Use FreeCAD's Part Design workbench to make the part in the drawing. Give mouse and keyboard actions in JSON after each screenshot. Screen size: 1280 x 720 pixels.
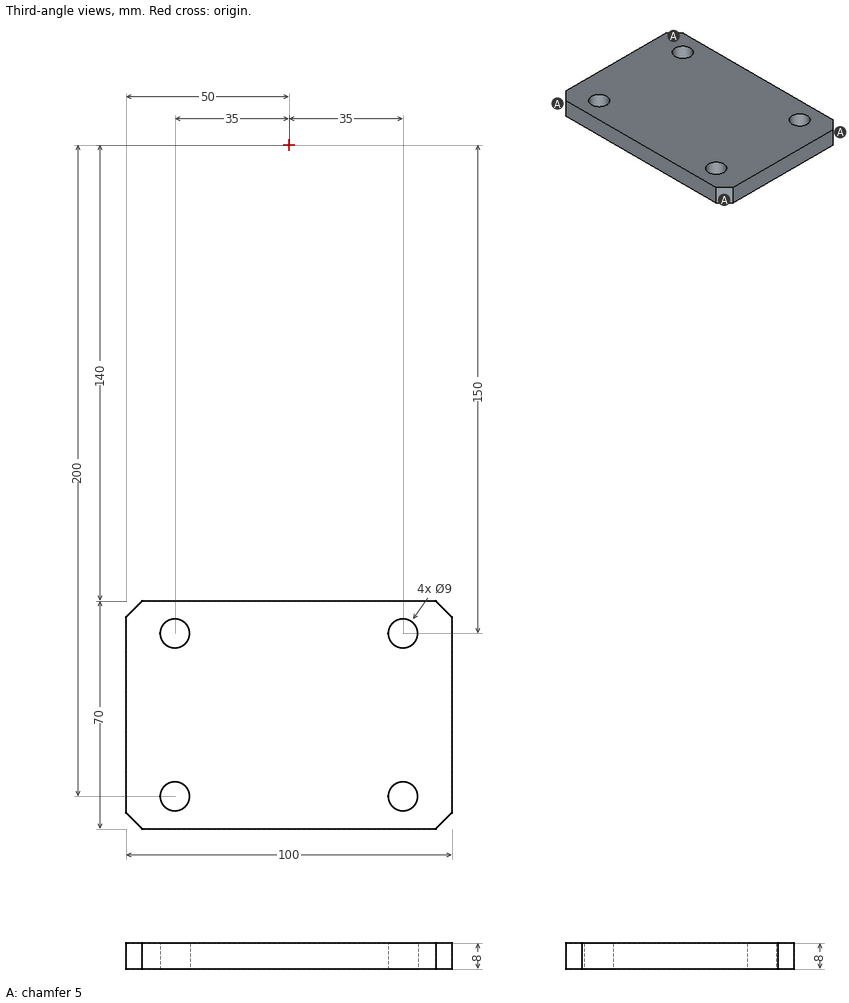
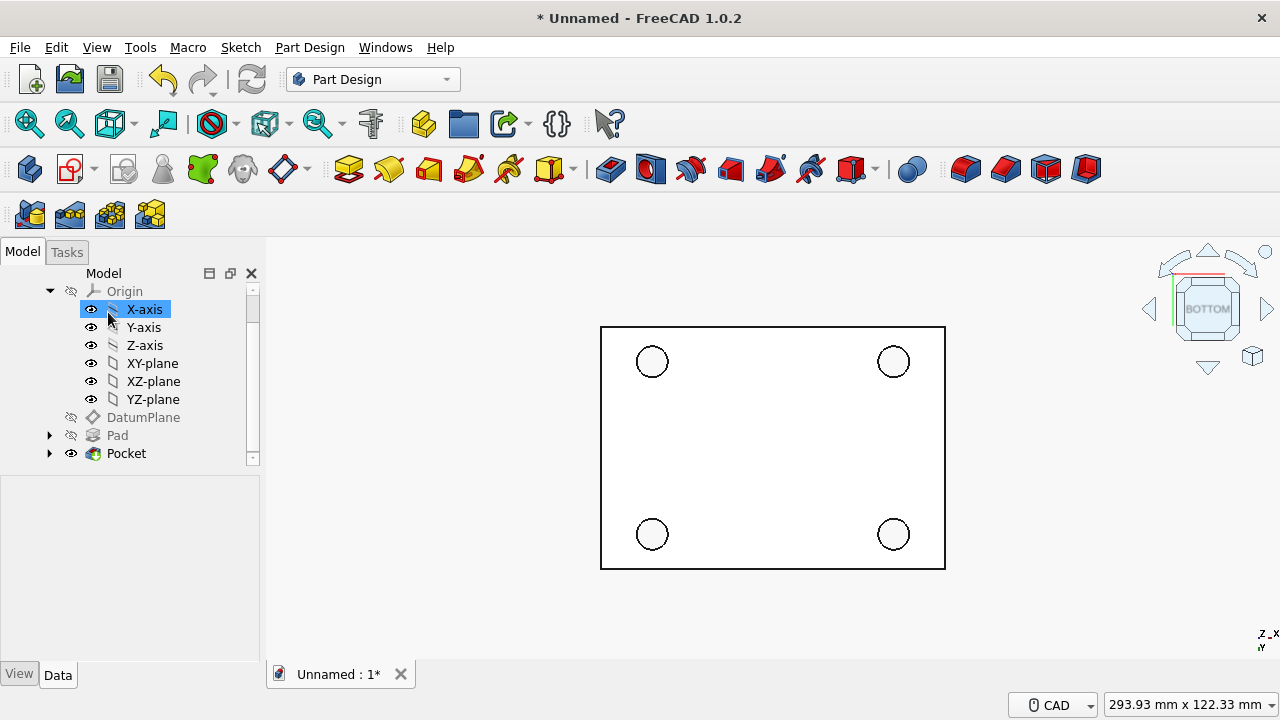
{"action": "key", "text": "0"}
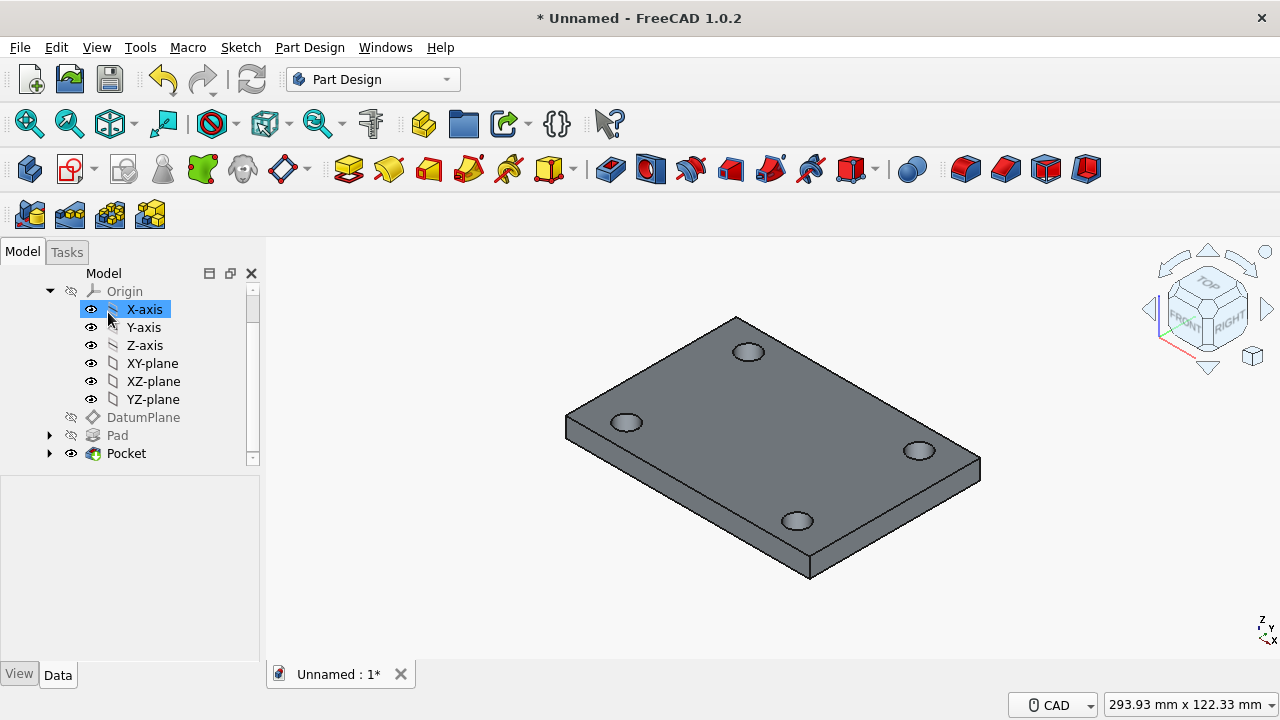
{"action": "left_click", "coordinate": [810, 567]}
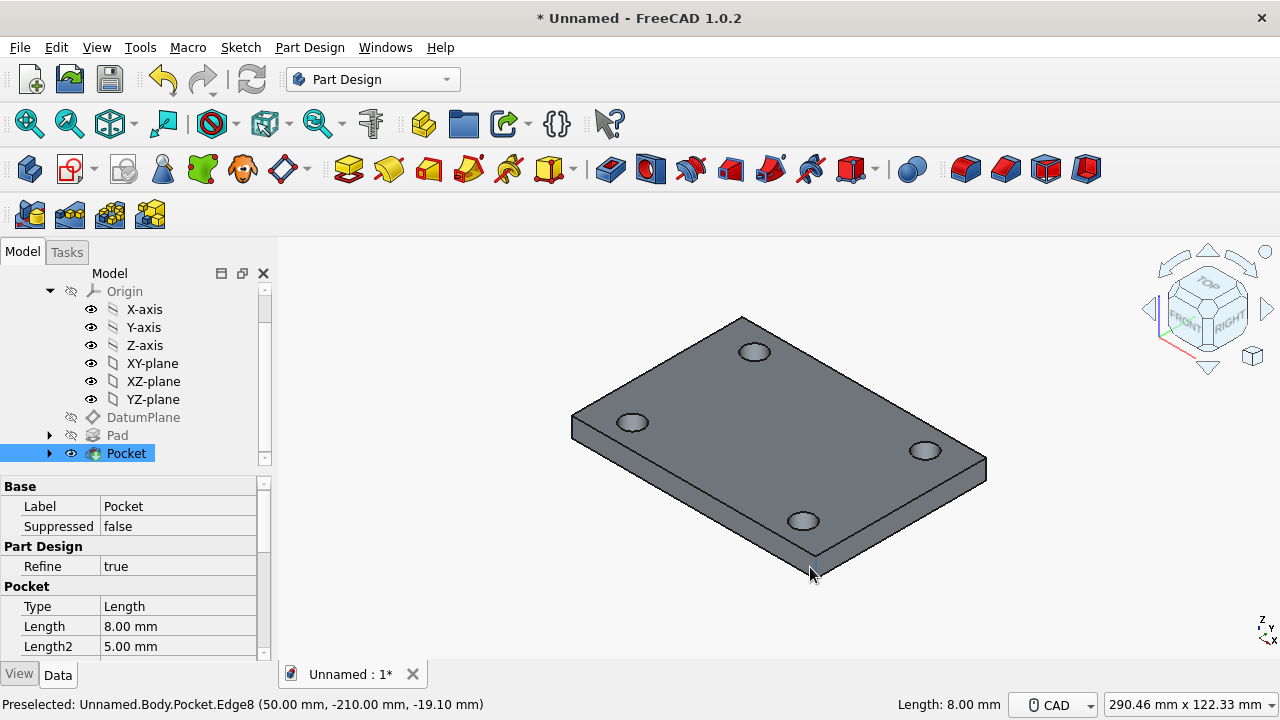
{"action": "key", "text": "2"}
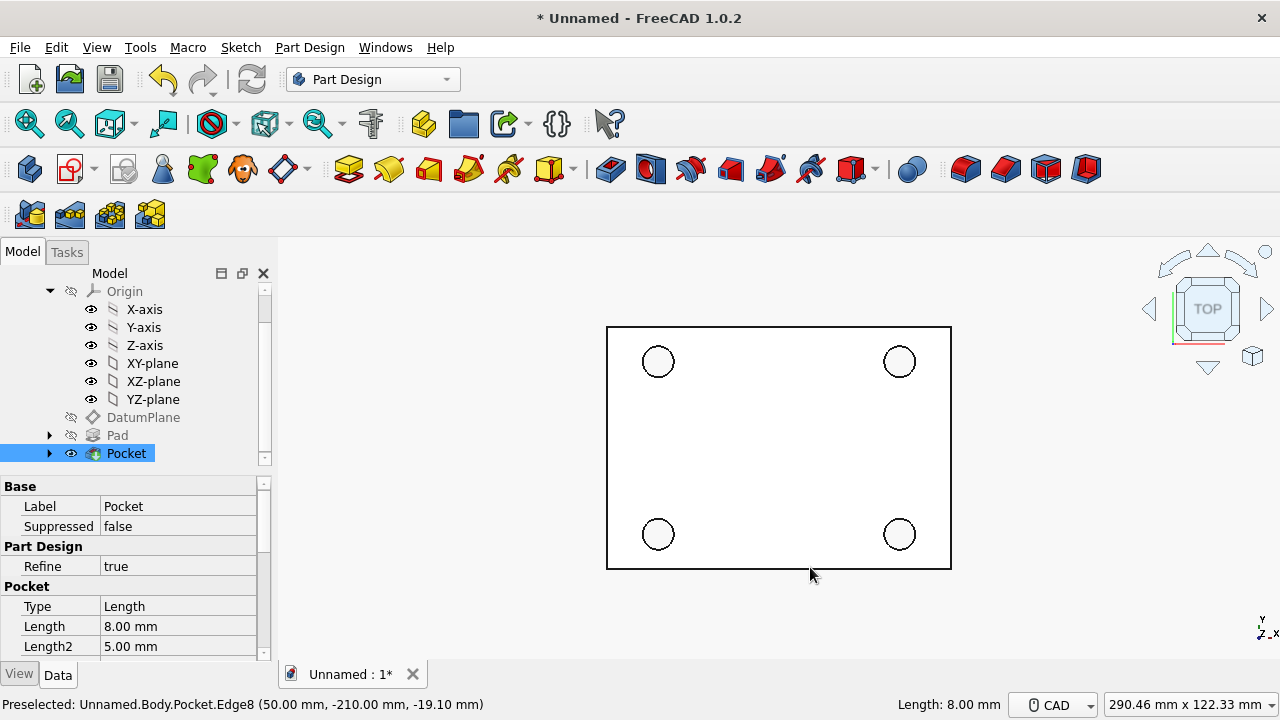
{"action": "key", "text": "1"}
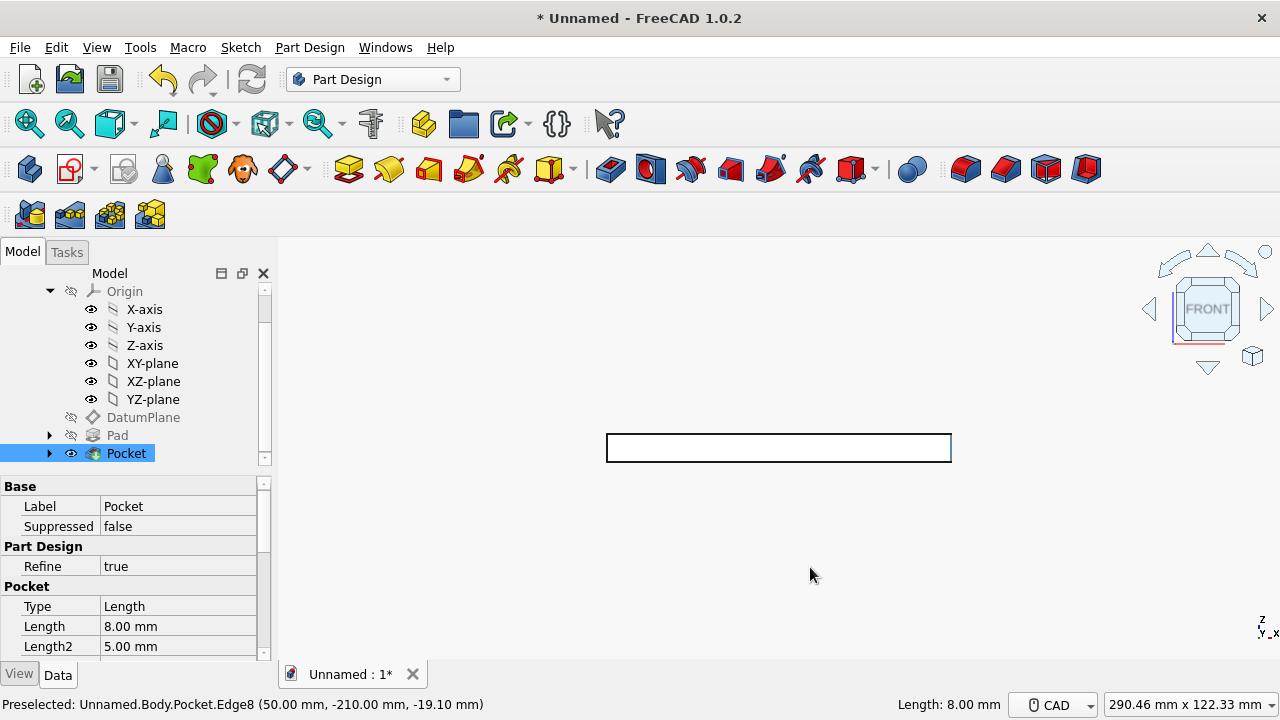
{"action": "left_click", "coordinate": [30, 124]}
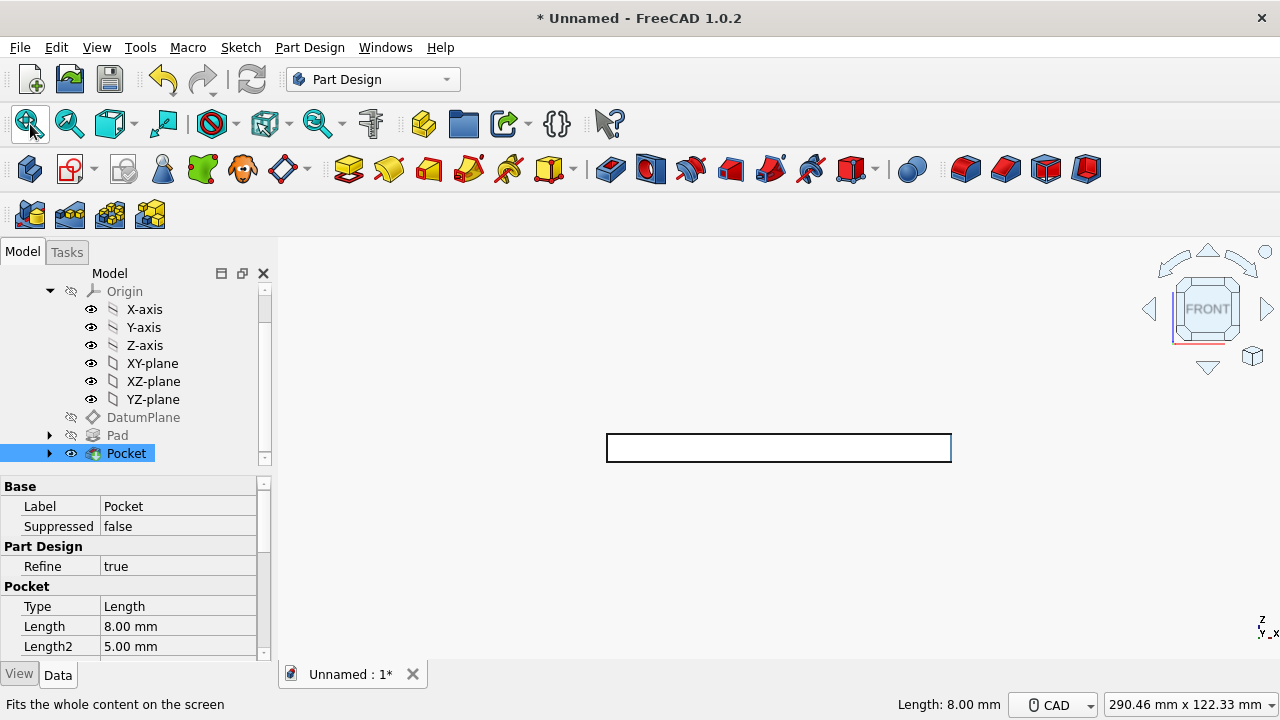
{"action": "left_click", "coordinate": [607, 447], "text": "ctrl"}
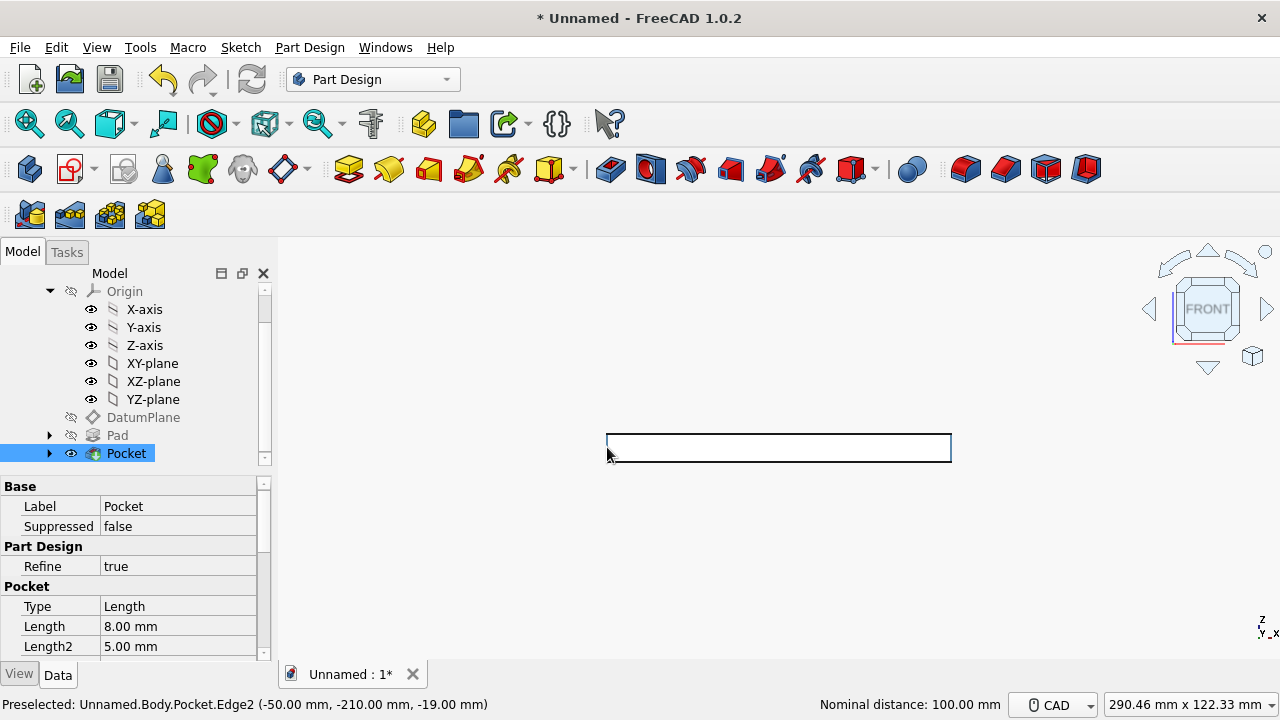
{"action": "key", "text": "3"}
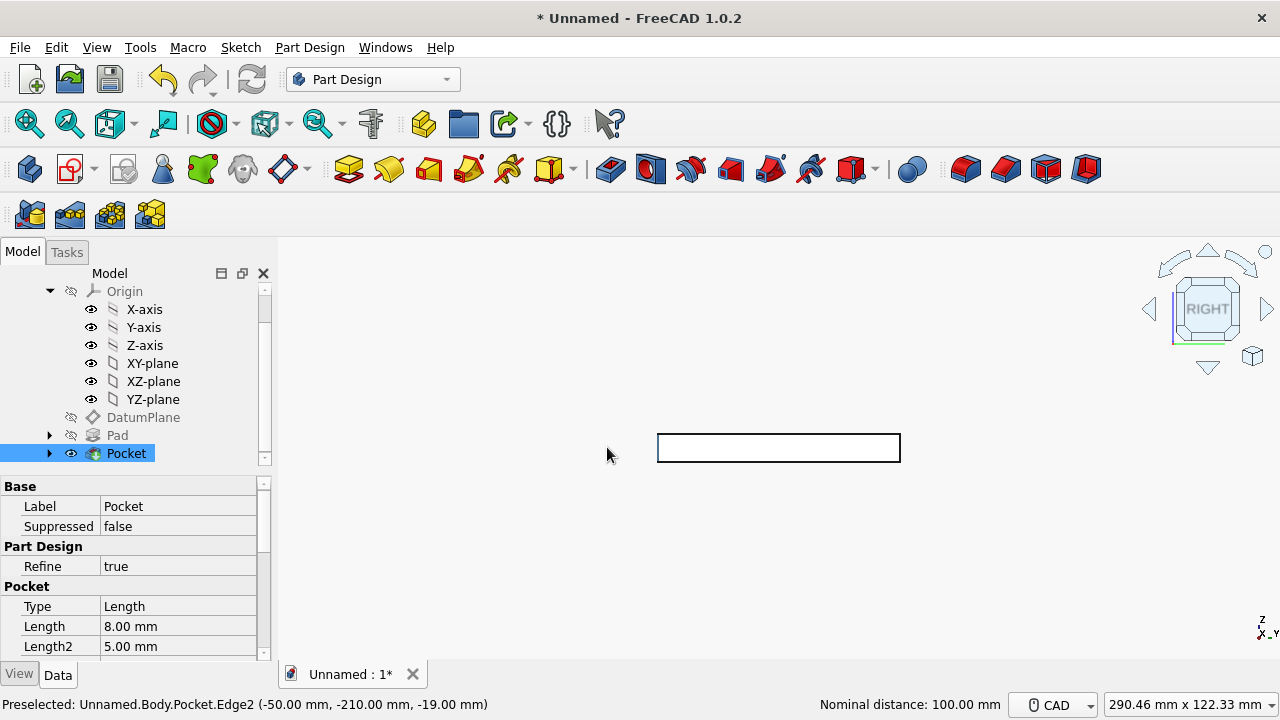
{"action": "left_click", "coordinate": [30, 124]}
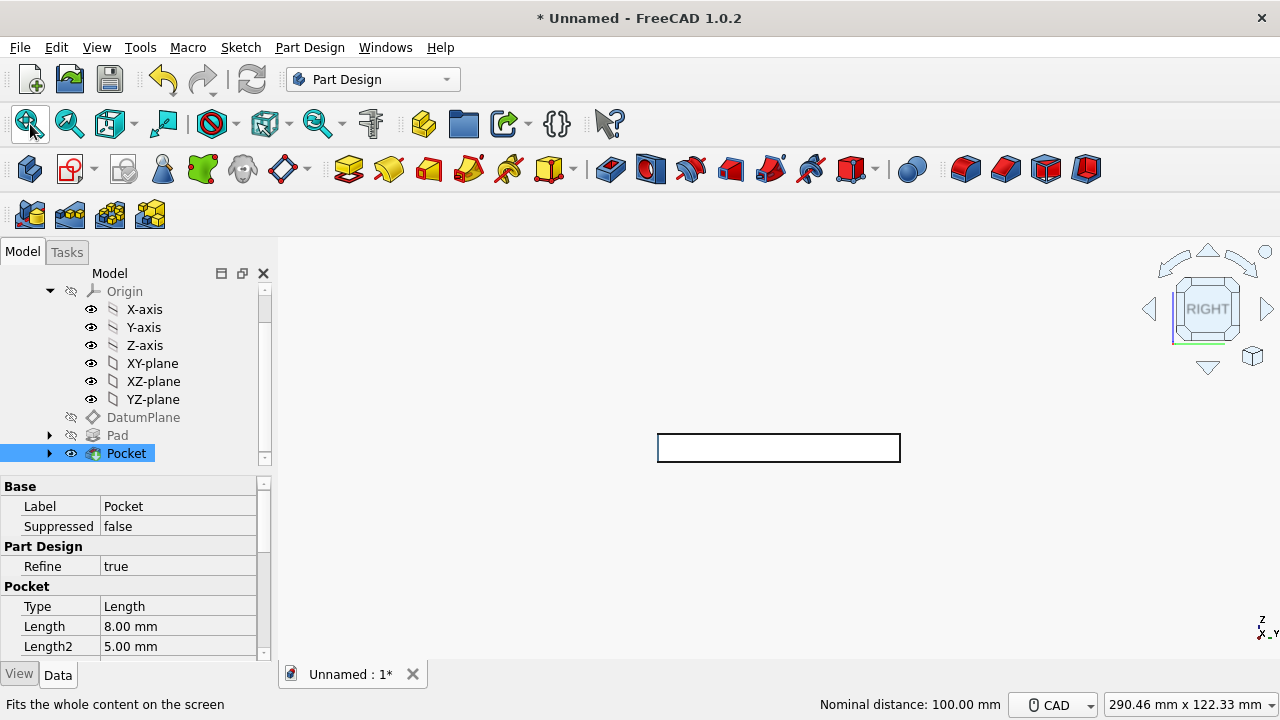
{"action": "left_click", "coordinate": [900, 447], "text": "ctrl"}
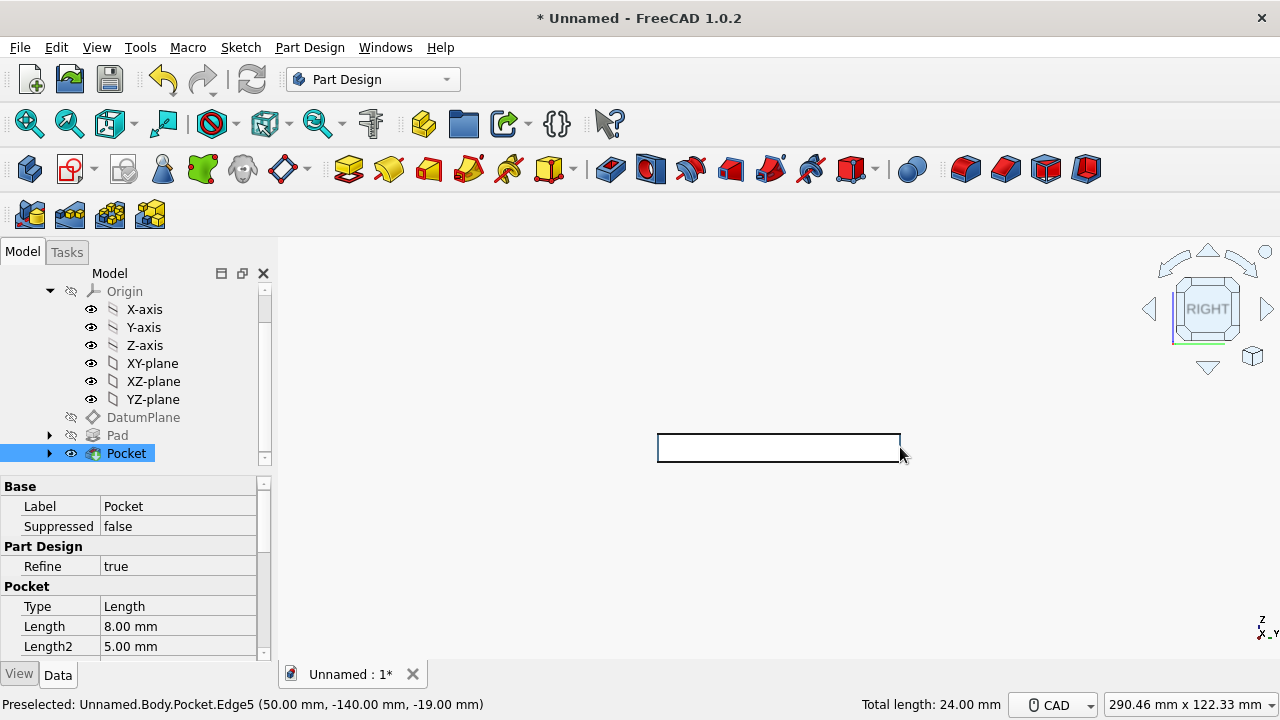
{"action": "key", "text": "5"}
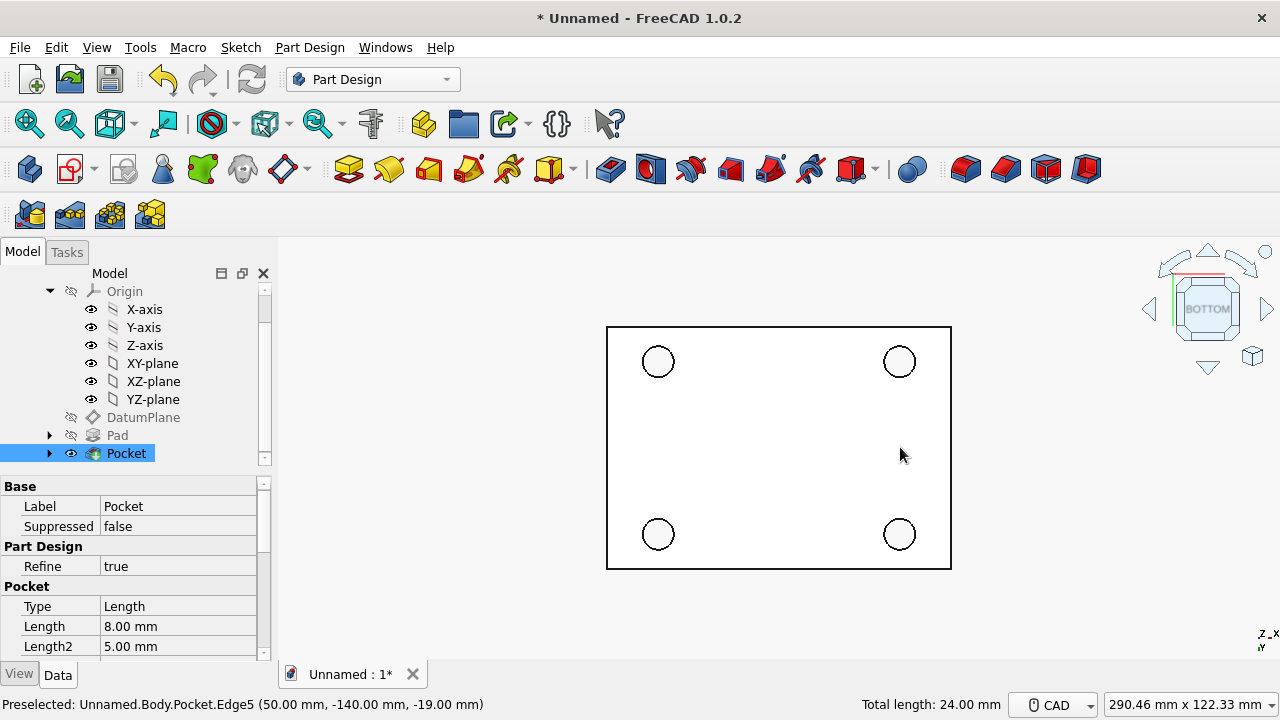
{"action": "key", "text": "4"}